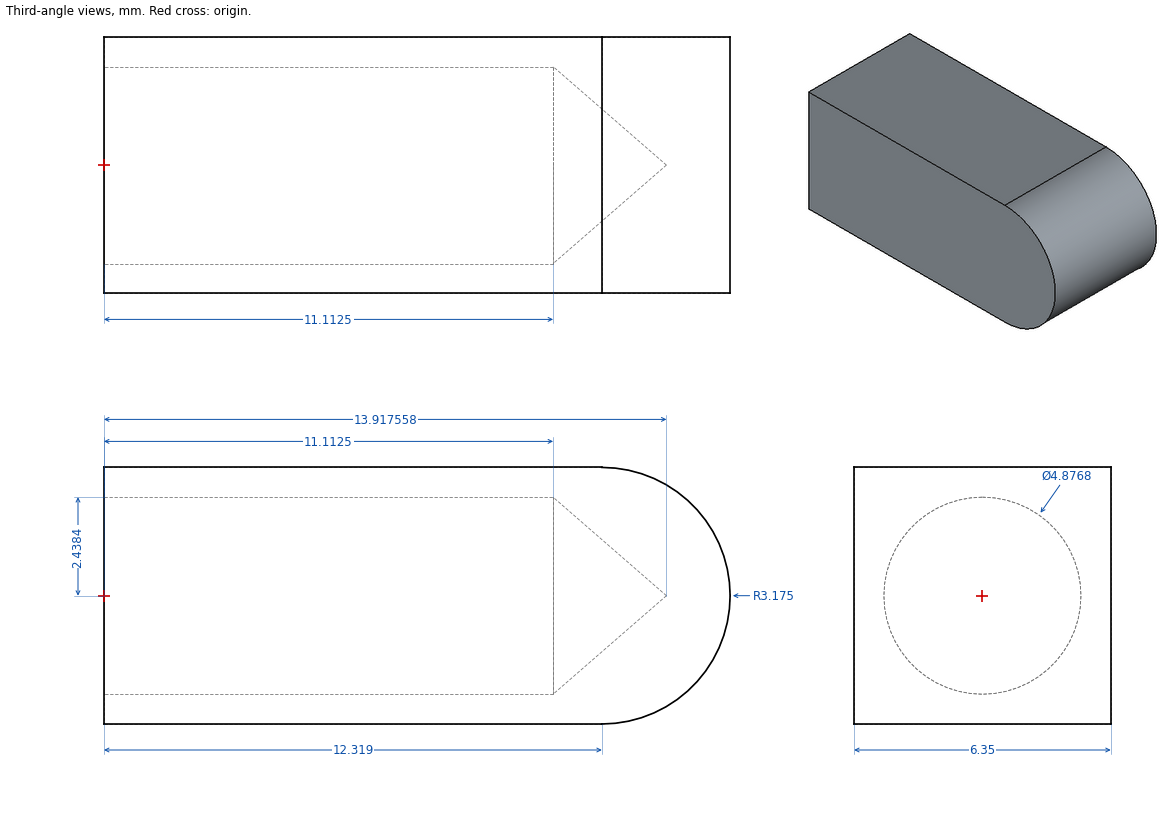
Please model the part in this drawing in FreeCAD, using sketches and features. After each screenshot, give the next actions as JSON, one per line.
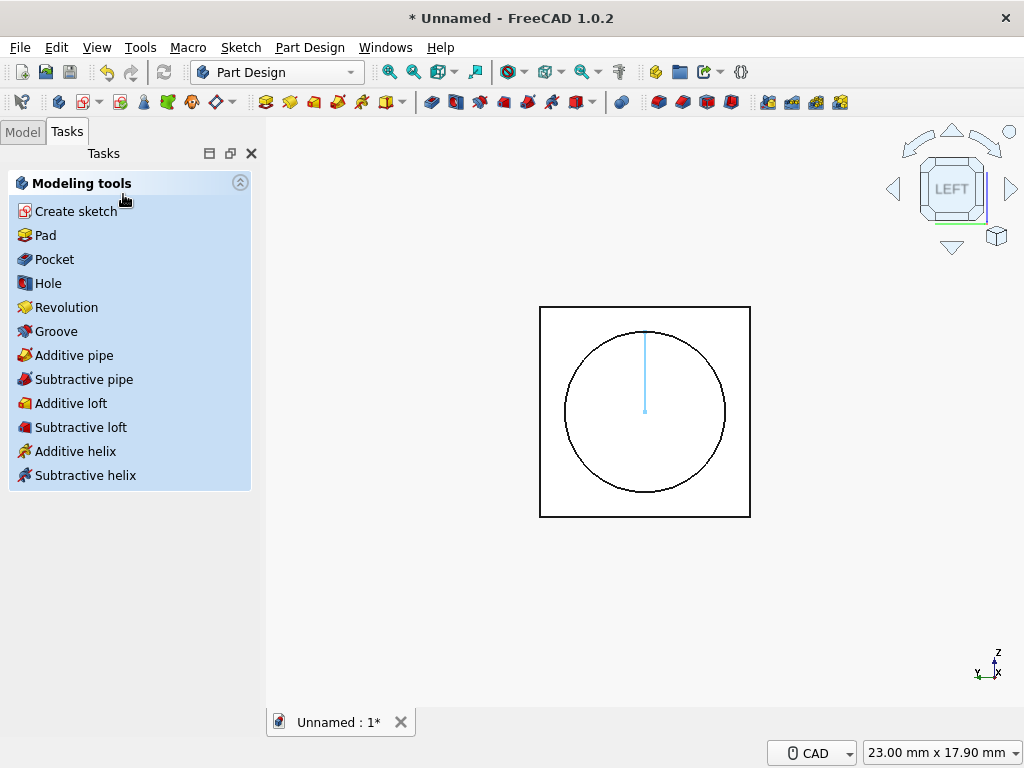
{"action": "left_click", "coordinate": [480, 102]}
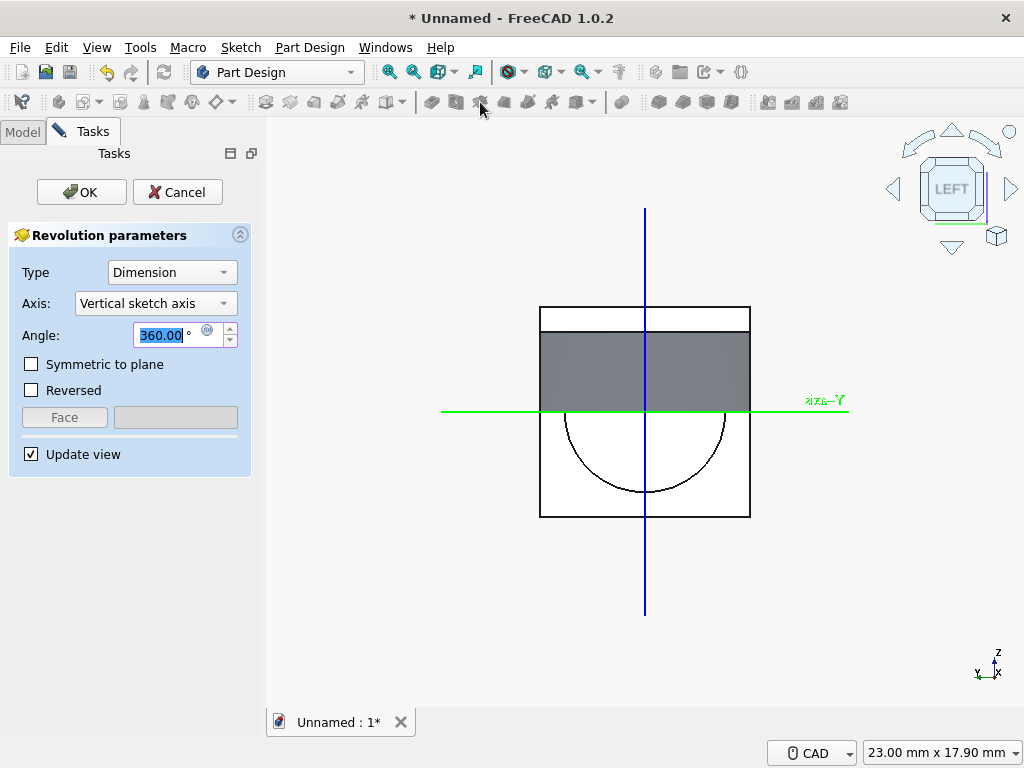
{"action": "left_click", "coordinate": [156, 304]}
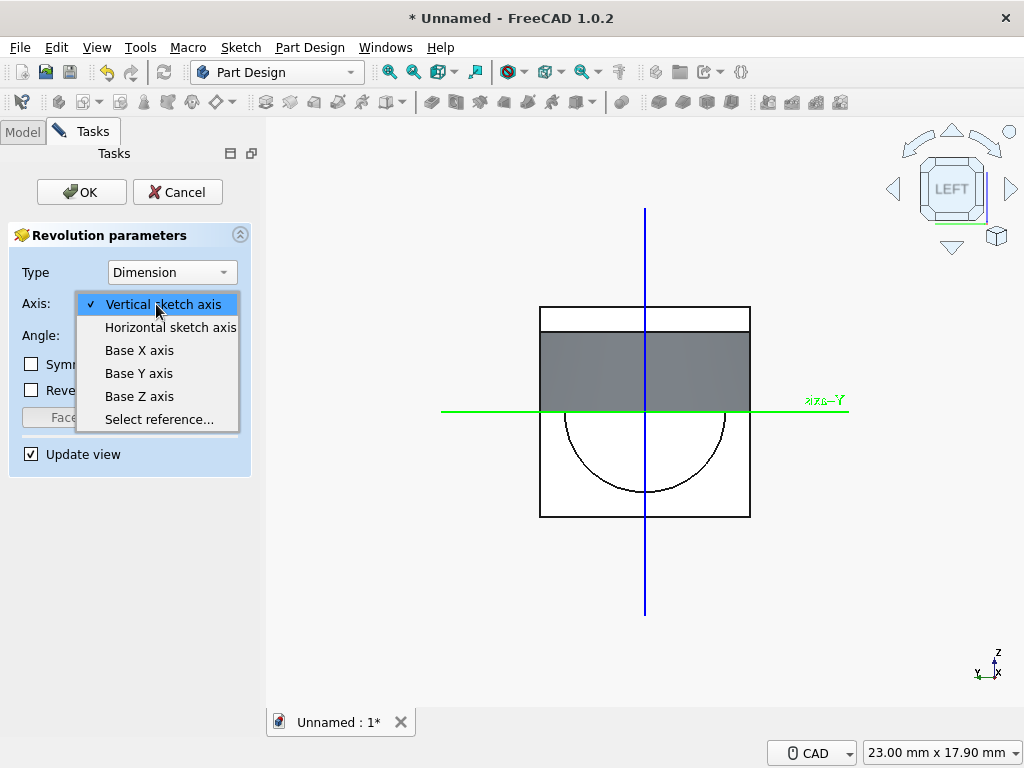
{"action": "left_click", "coordinate": [156, 328]}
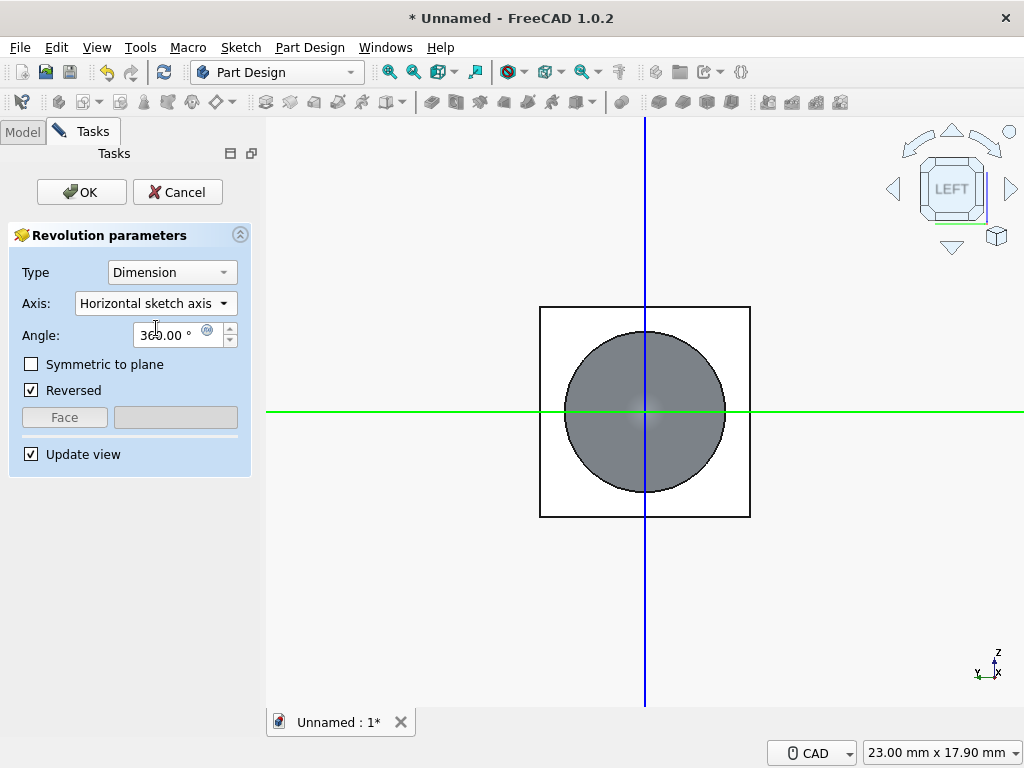
{"action": "left_click", "coordinate": [82, 192]}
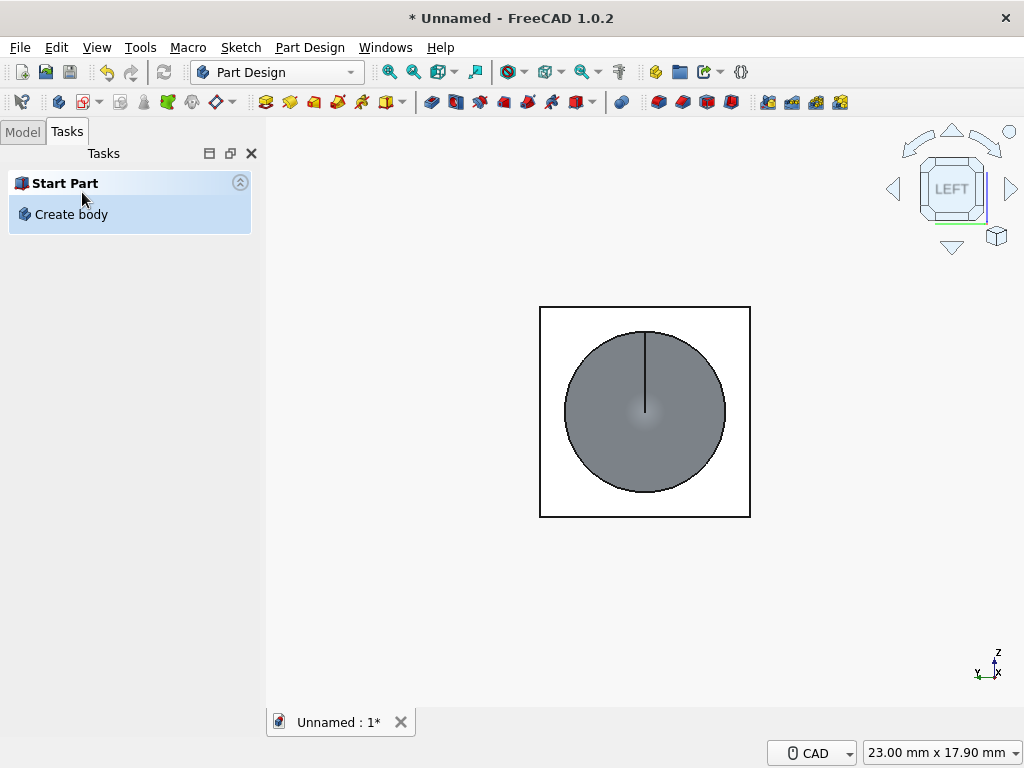
{"action": "key", "text": "0"}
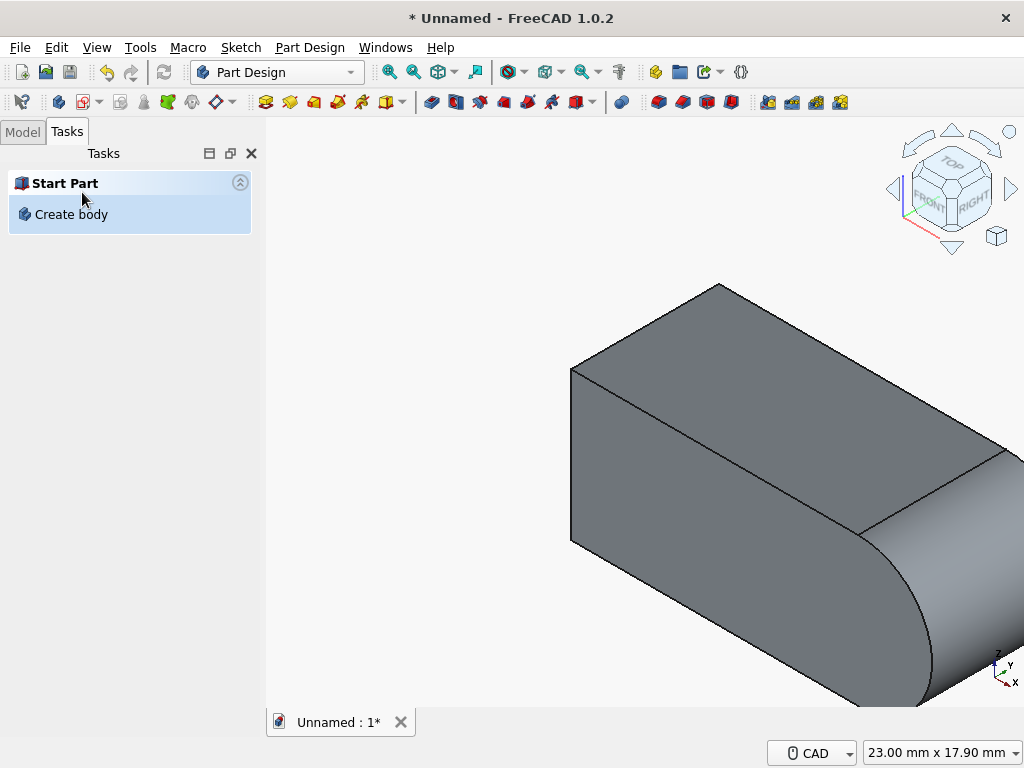
{"action": "key", "text": "v f"}